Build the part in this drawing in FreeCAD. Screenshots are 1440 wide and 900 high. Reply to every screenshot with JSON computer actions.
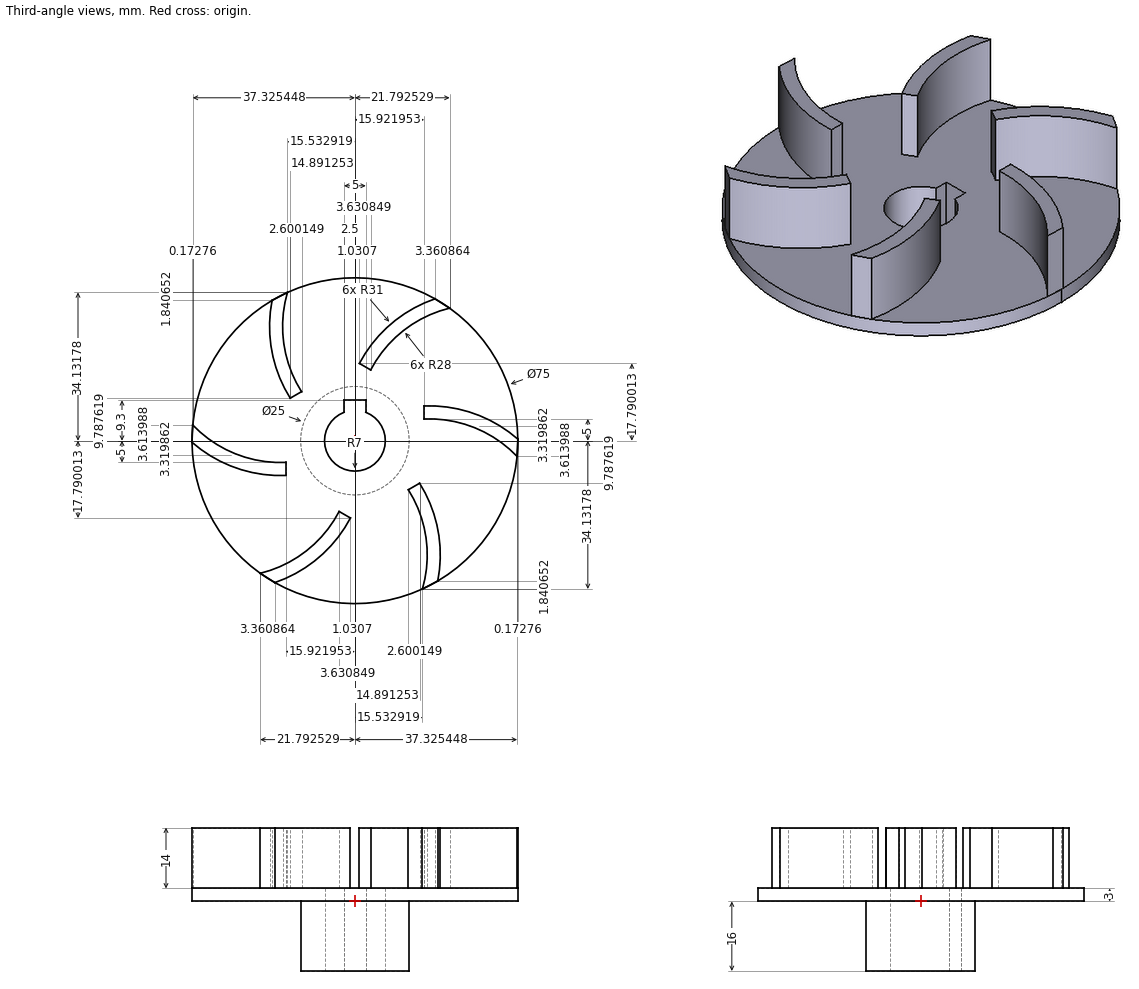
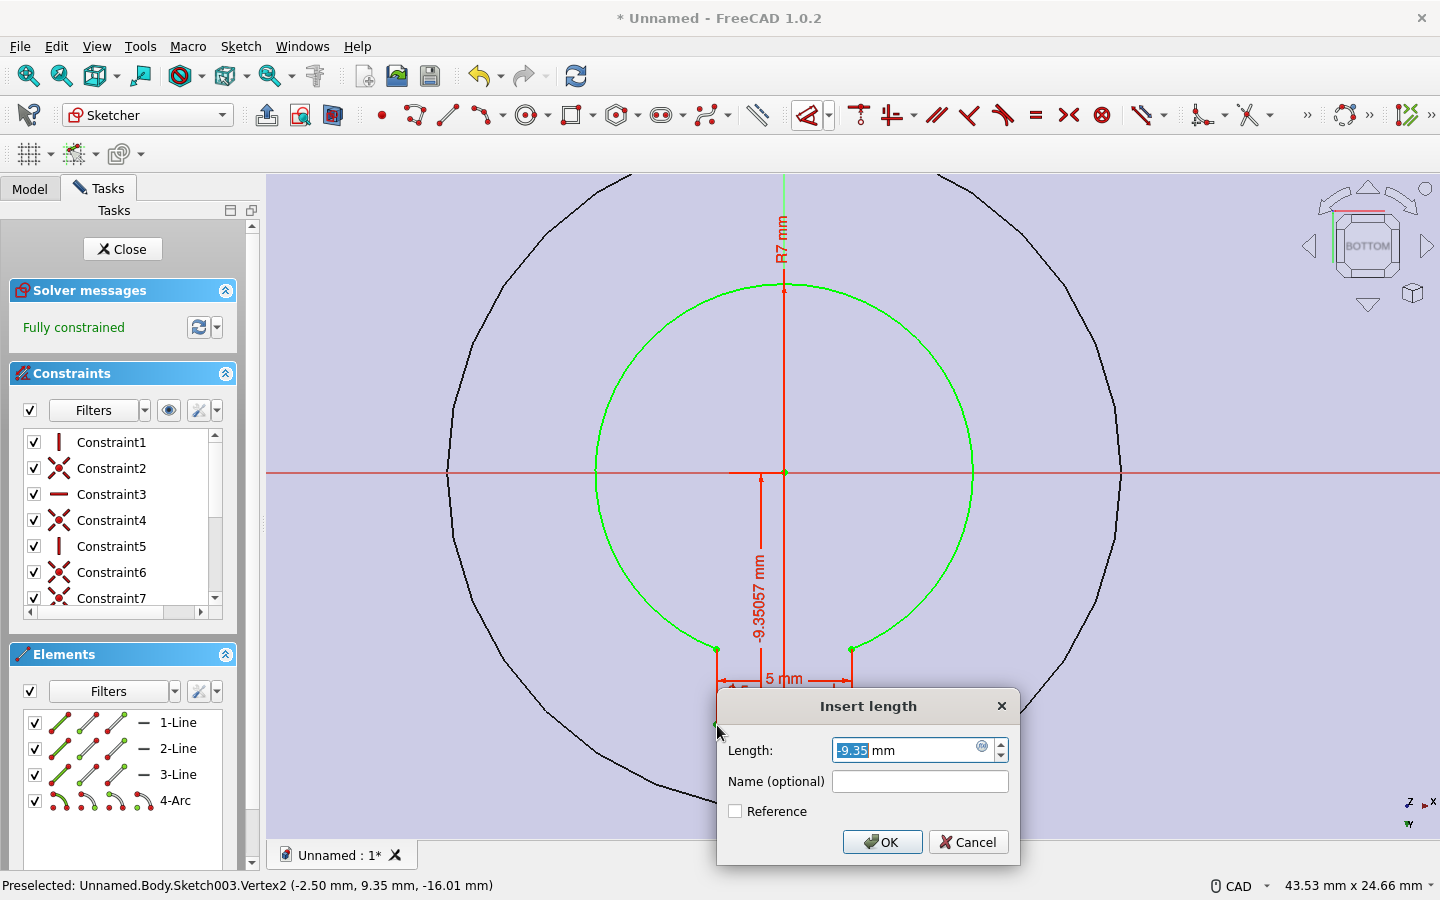
{"action": "type", "text": "-9.3"}
{"action": "key", "text": "Return"}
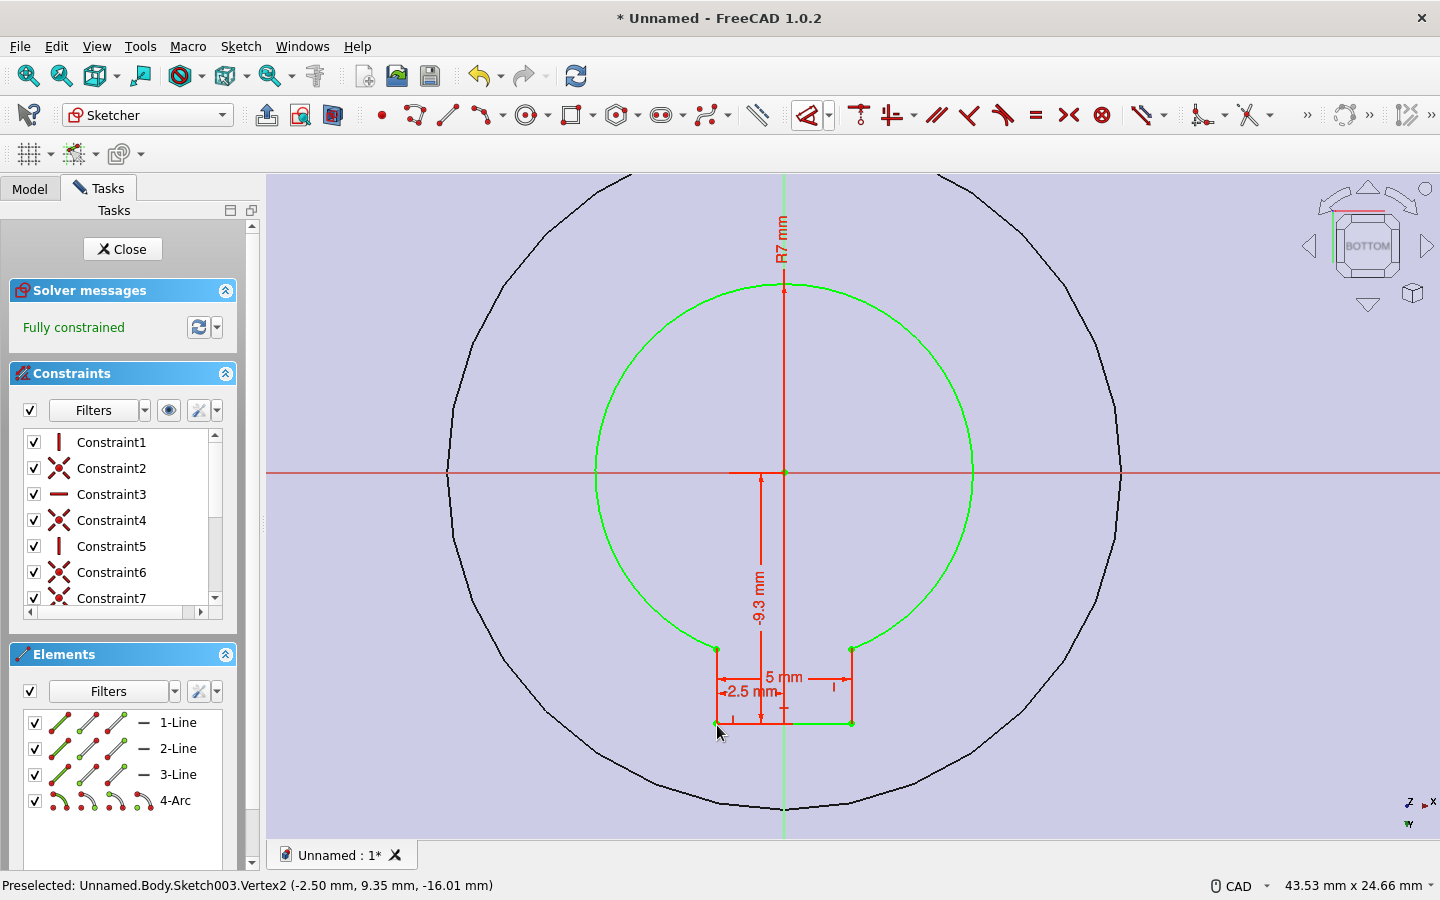
{"action": "left_click", "coordinate": [123, 249]}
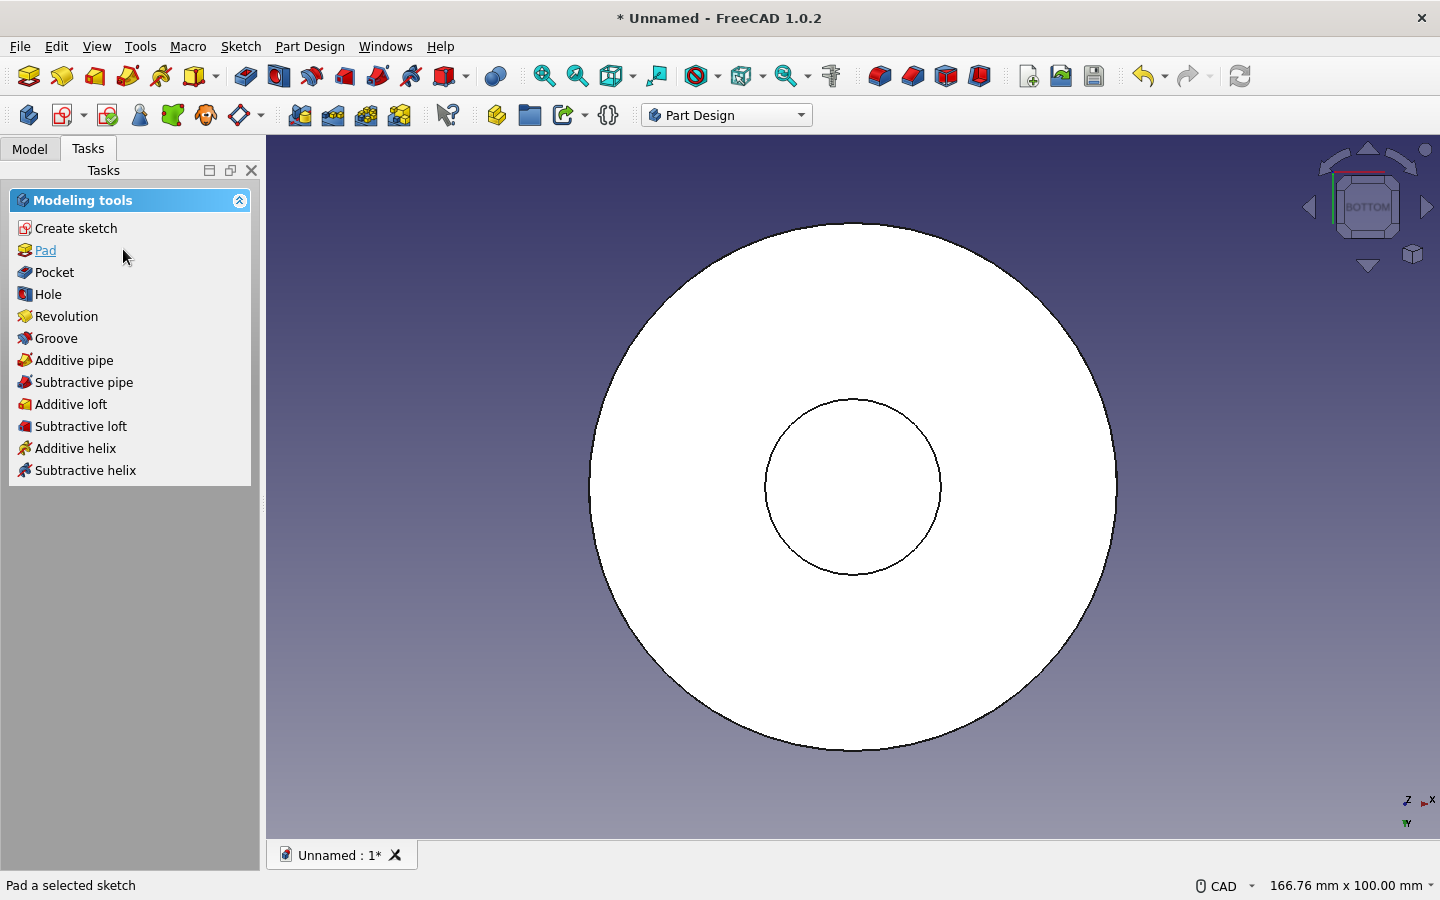
{"action": "left_click", "coordinate": [246, 76]}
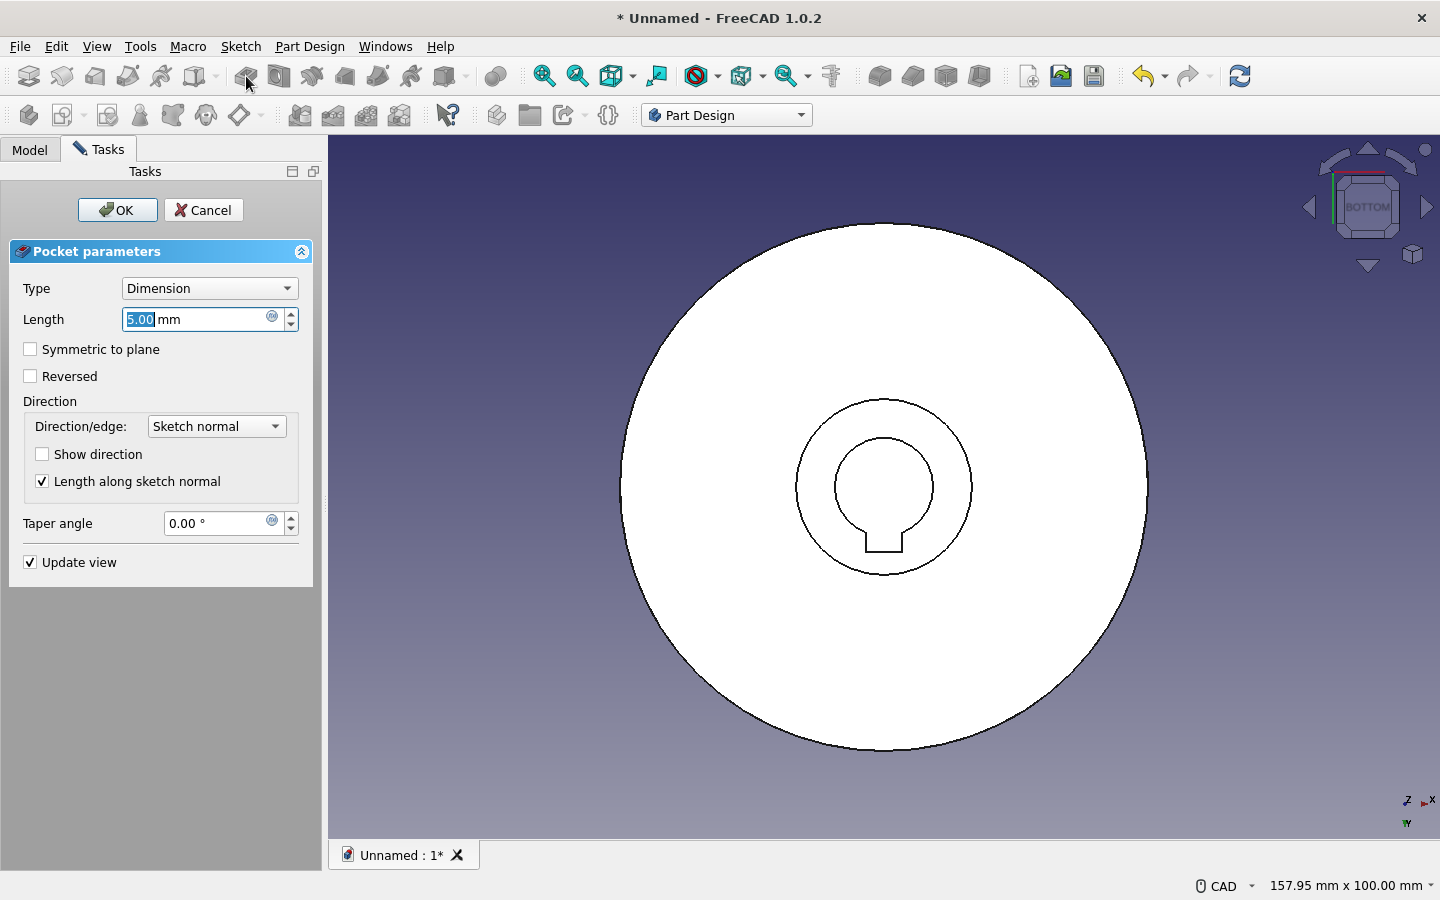
{"action": "left_click", "coordinate": [210, 288]}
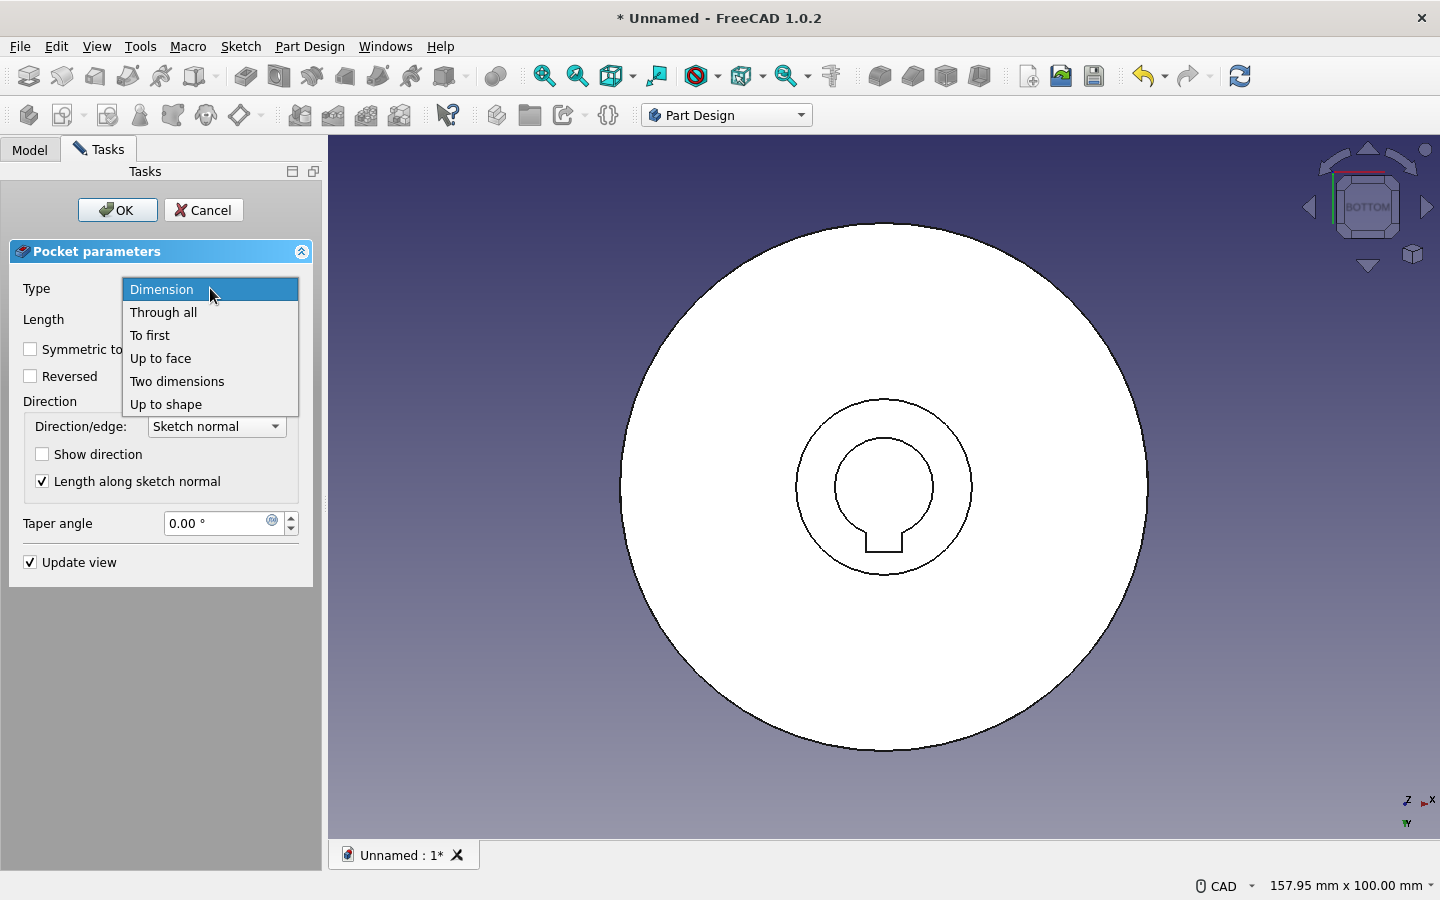
{"action": "left_click", "coordinate": [208, 312]}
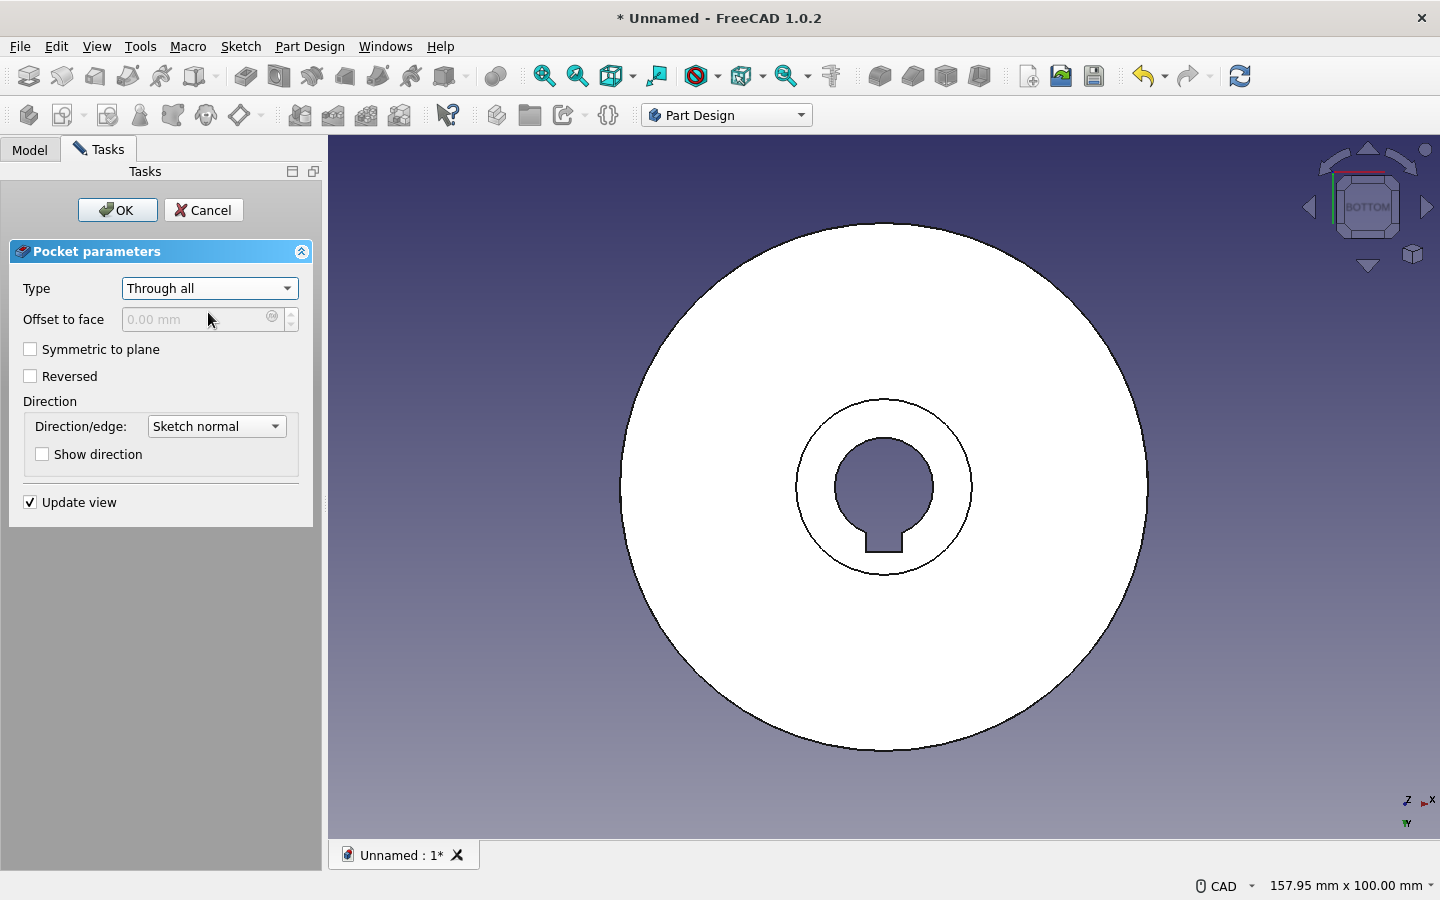
{"action": "left_click", "coordinate": [118, 210]}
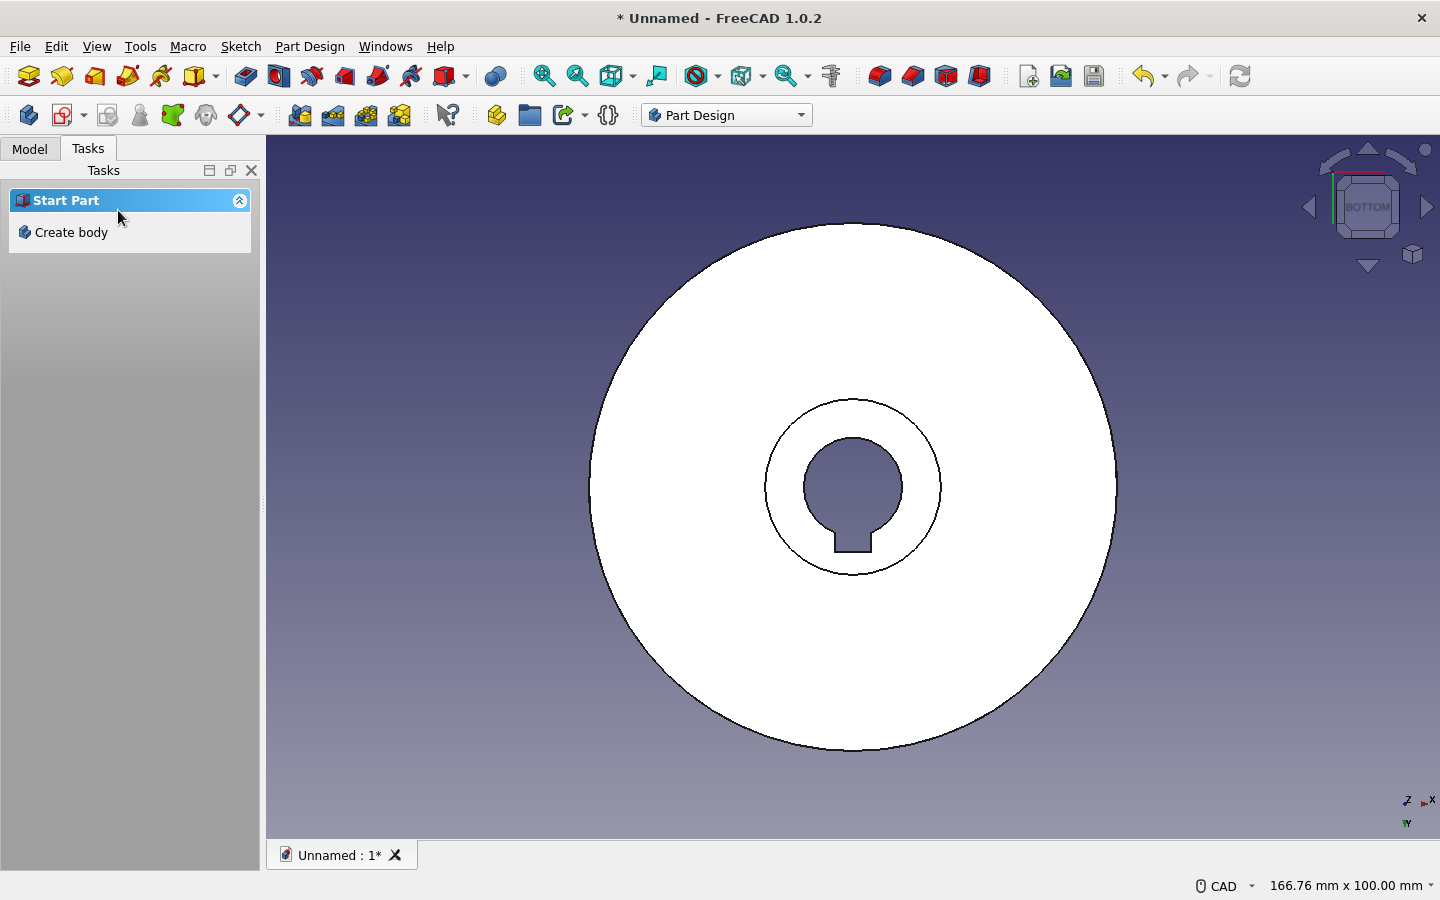
{"action": "key", "text": "0"}